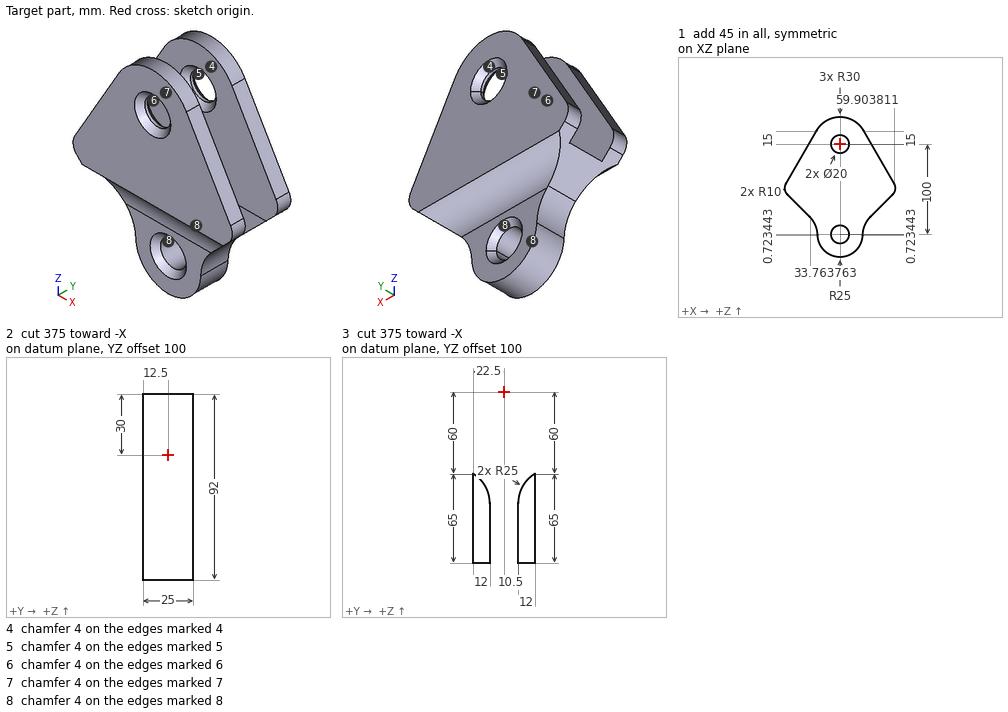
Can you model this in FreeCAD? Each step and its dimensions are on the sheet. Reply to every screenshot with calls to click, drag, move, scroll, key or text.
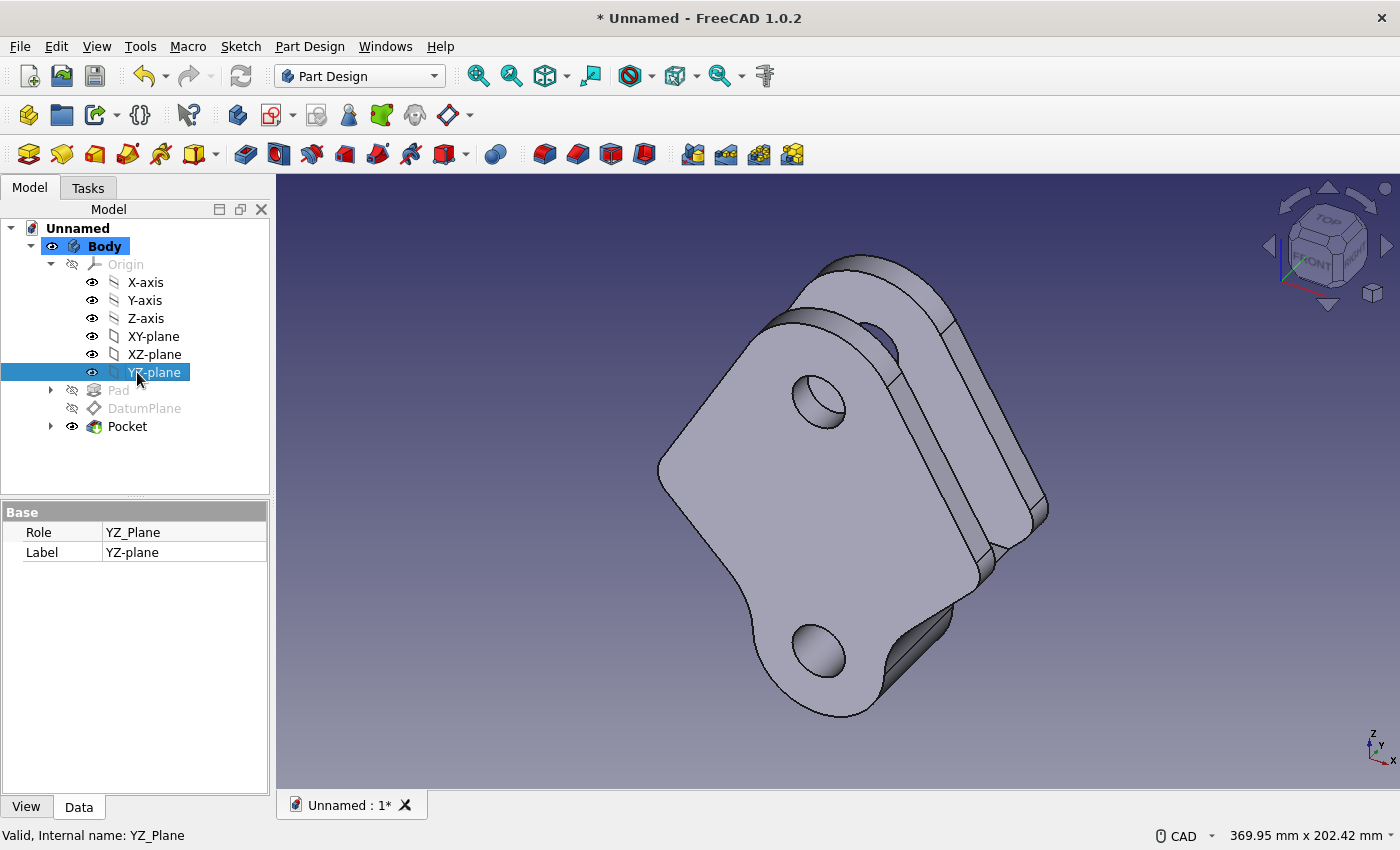
click(448, 116)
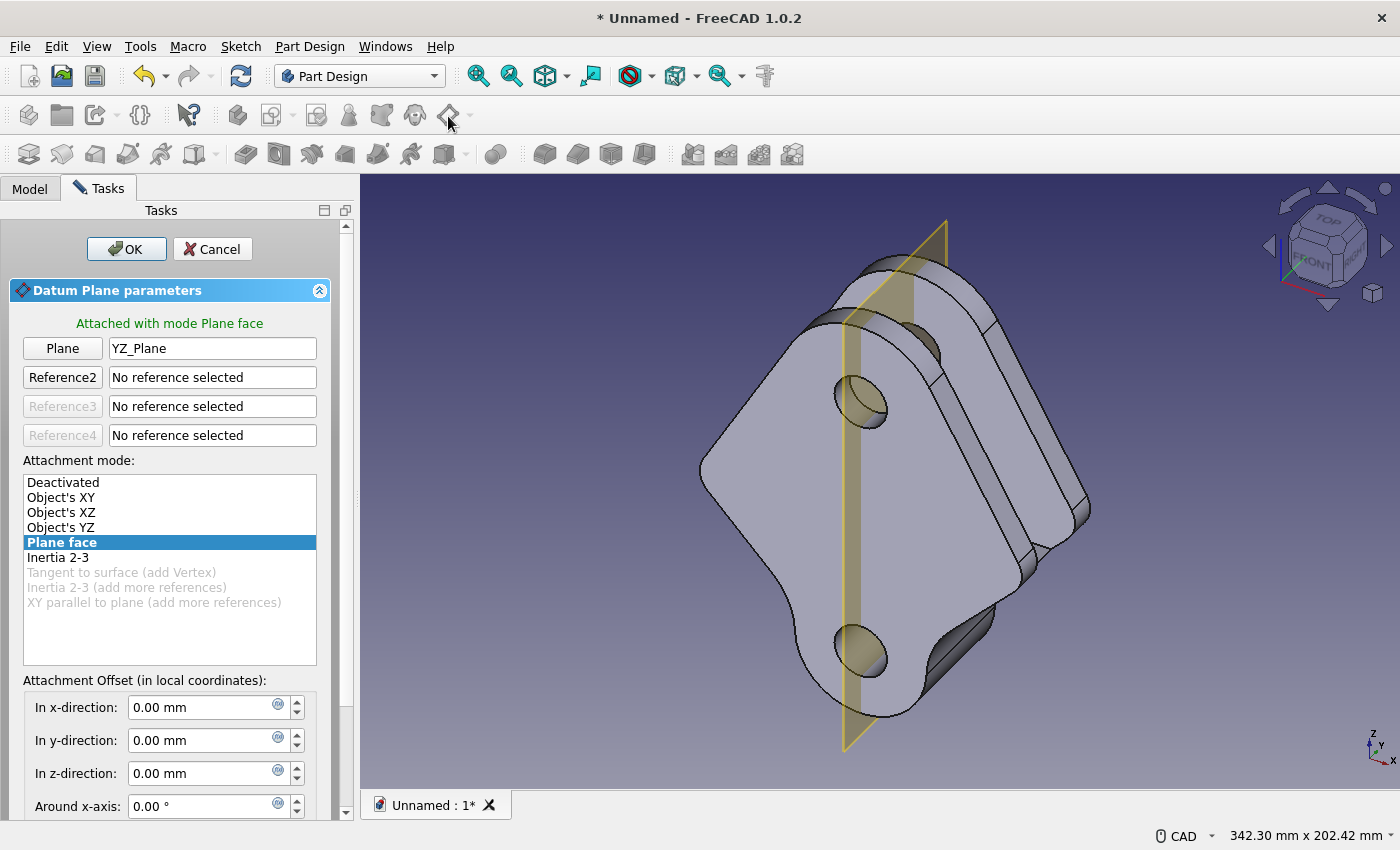
triple_click(210, 774)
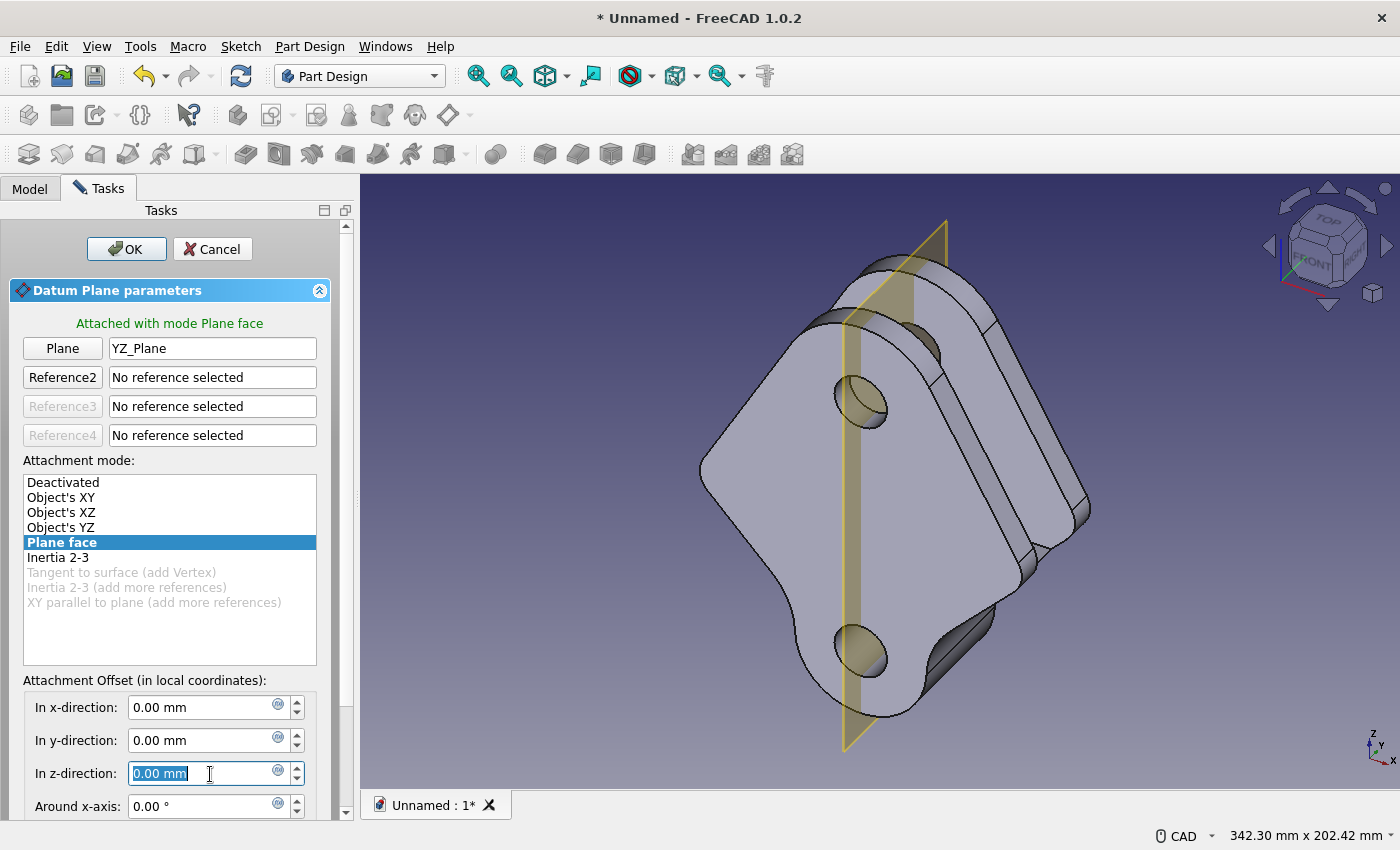
text(100)
key(Tab)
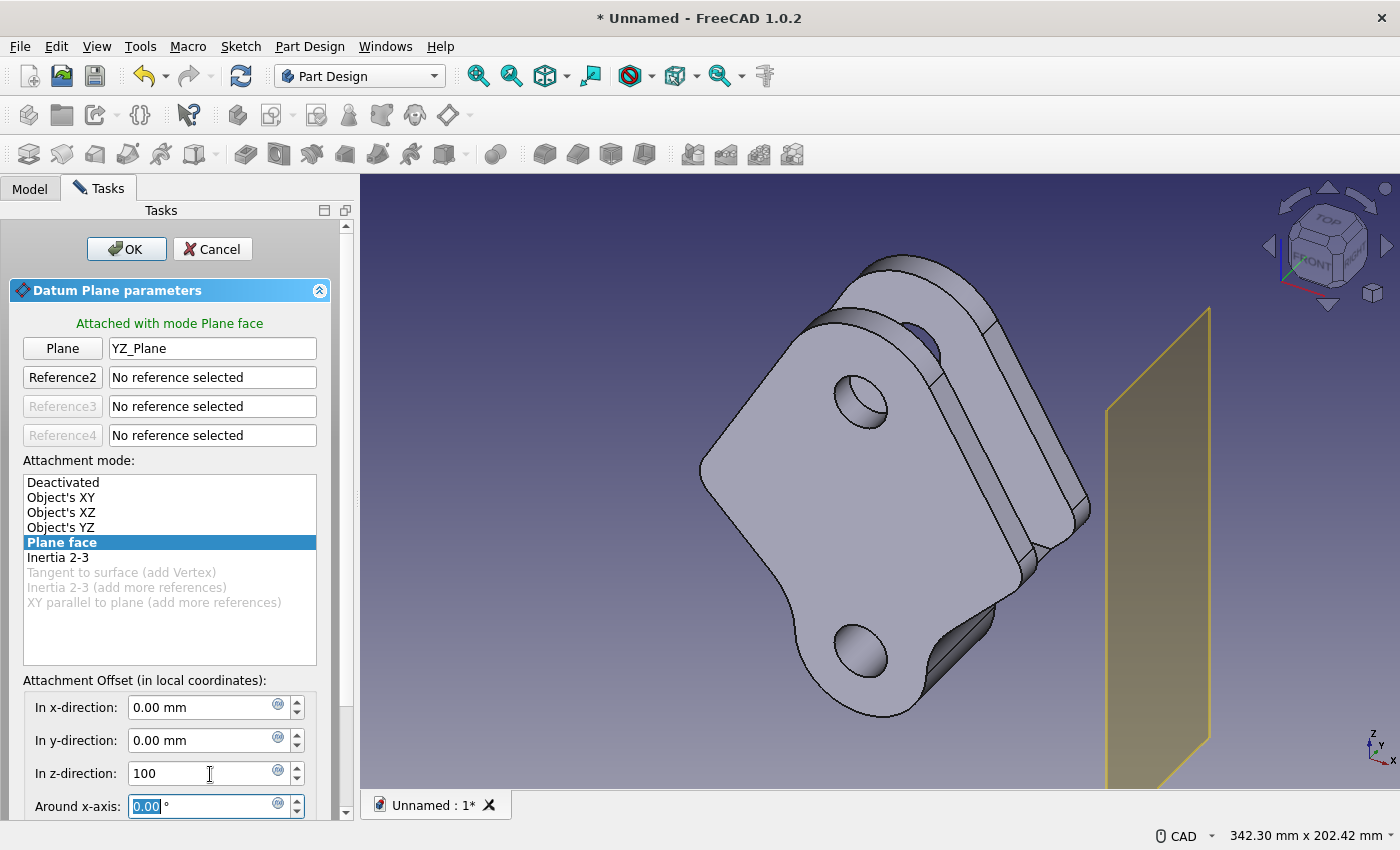
click(127, 249)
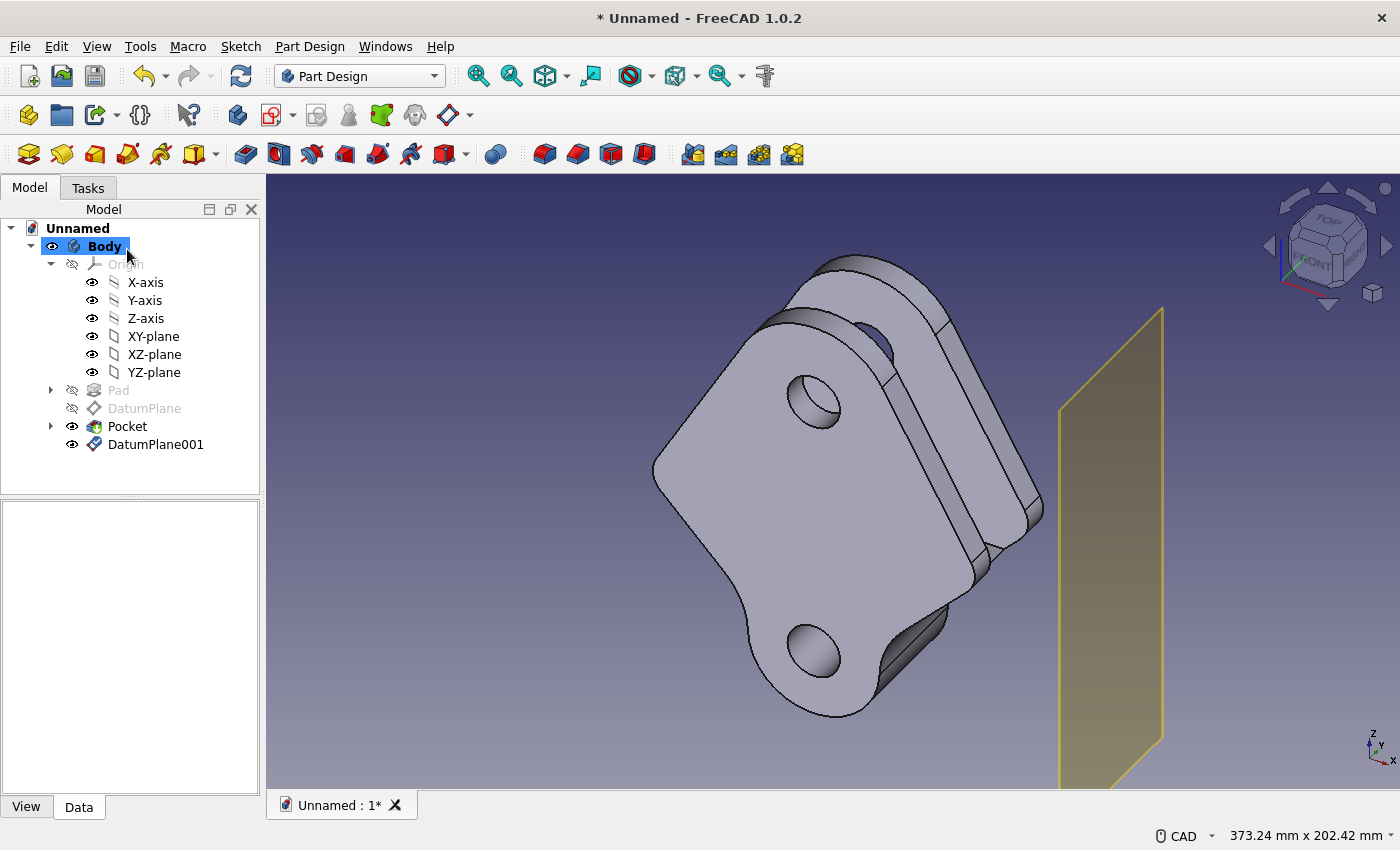
click(117, 444)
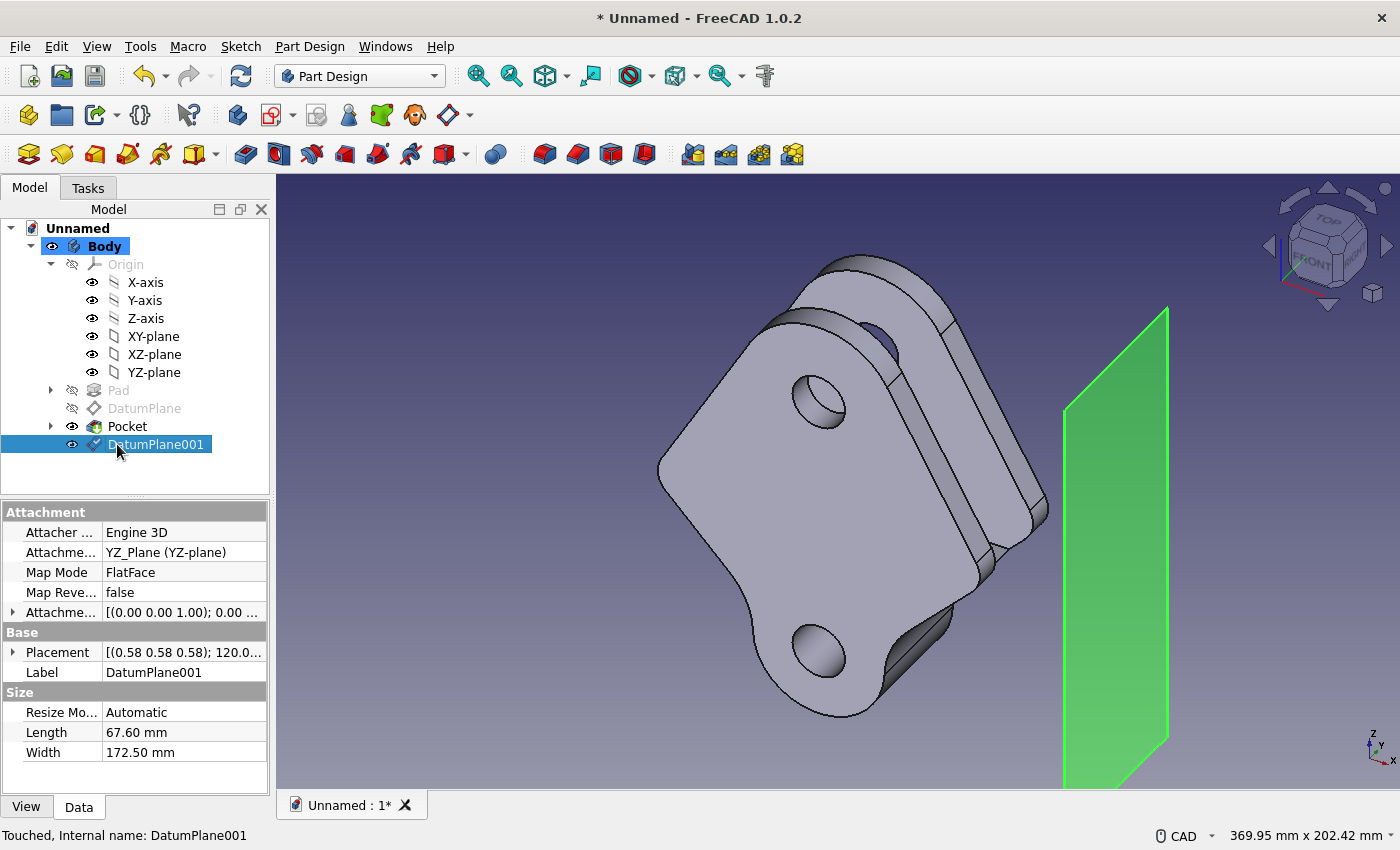
click(270, 116)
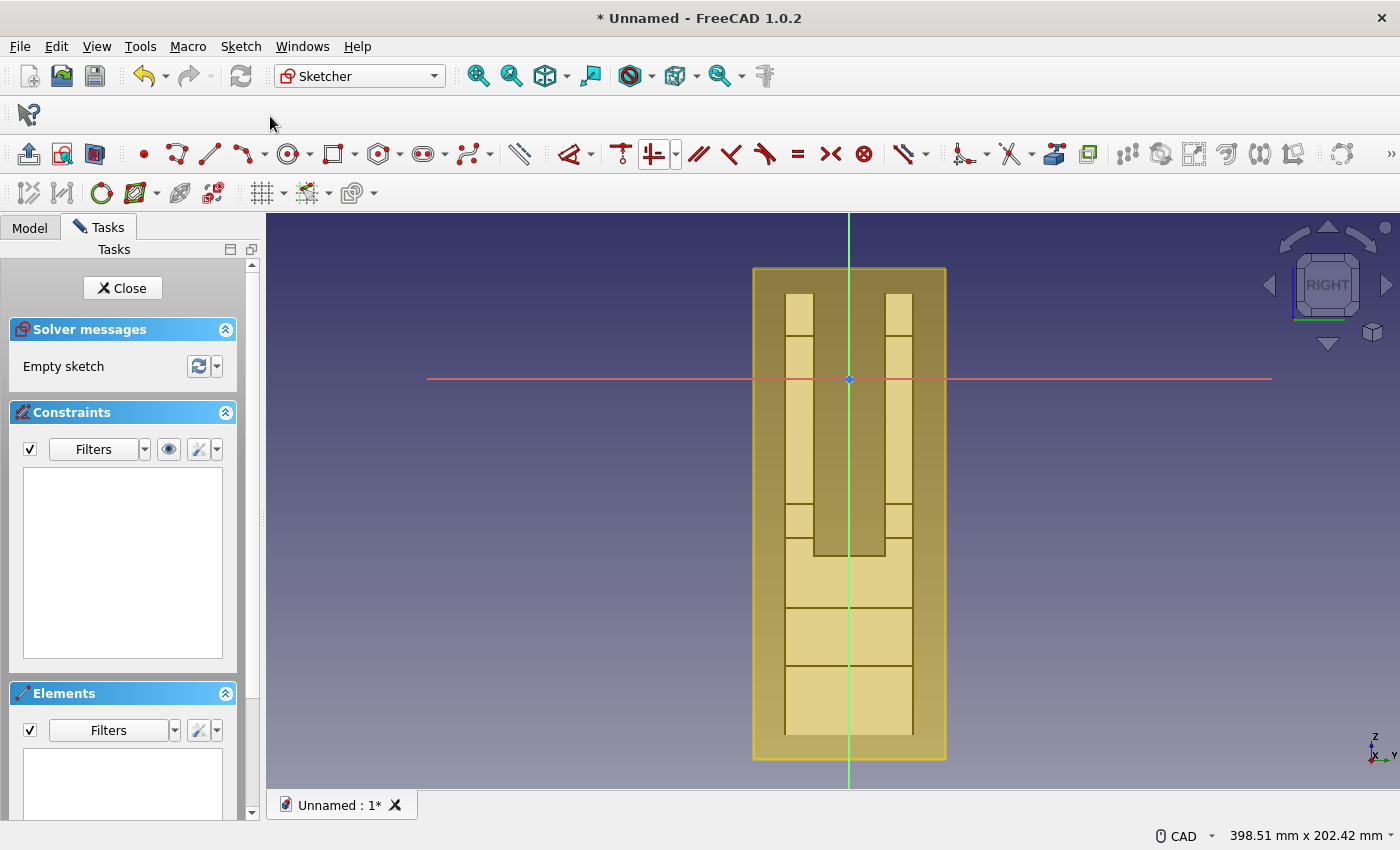
click(177, 154)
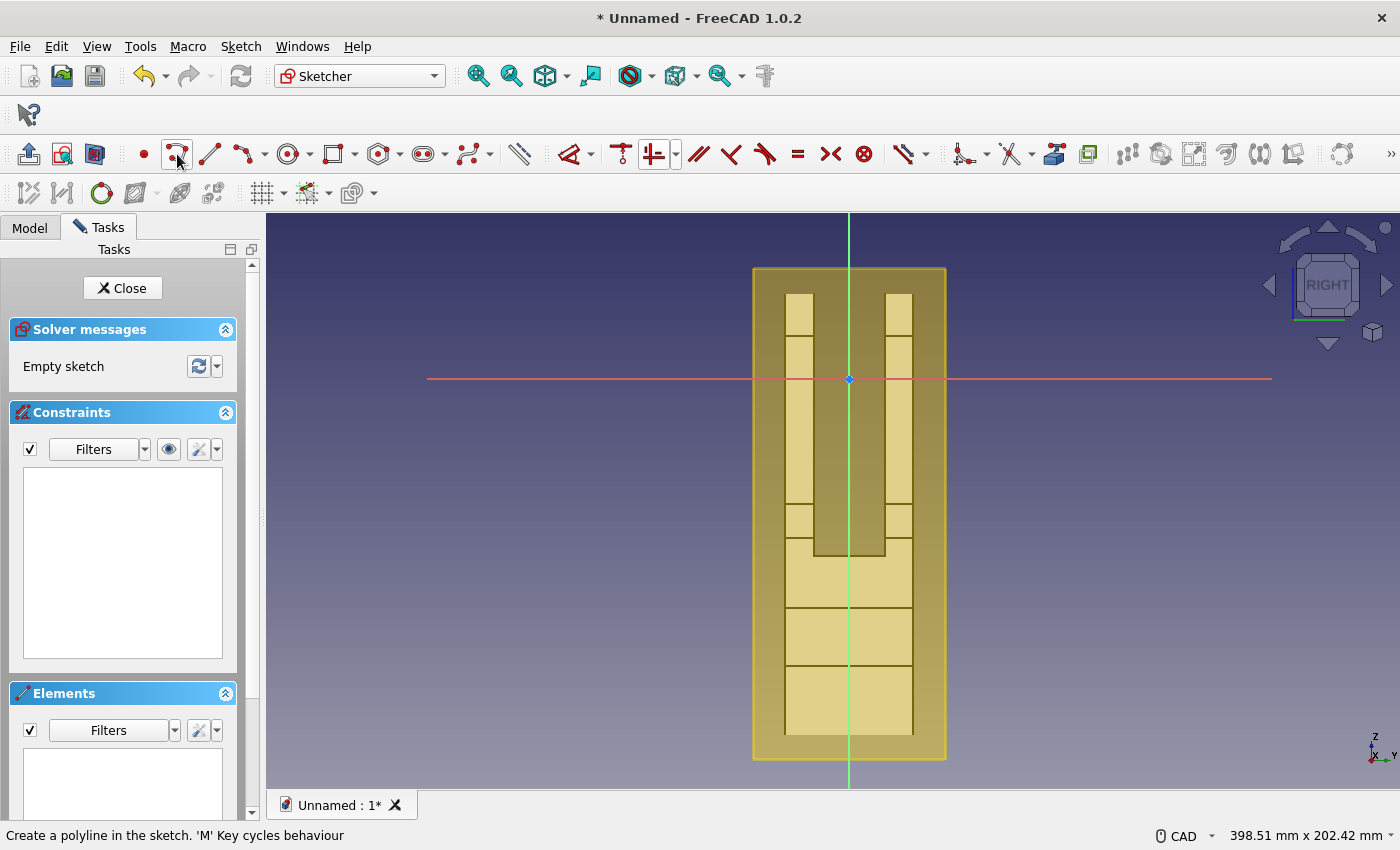
click(879, 611)
click(879, 735)
click(913, 735)
click(913, 550)
right_click(913, 550)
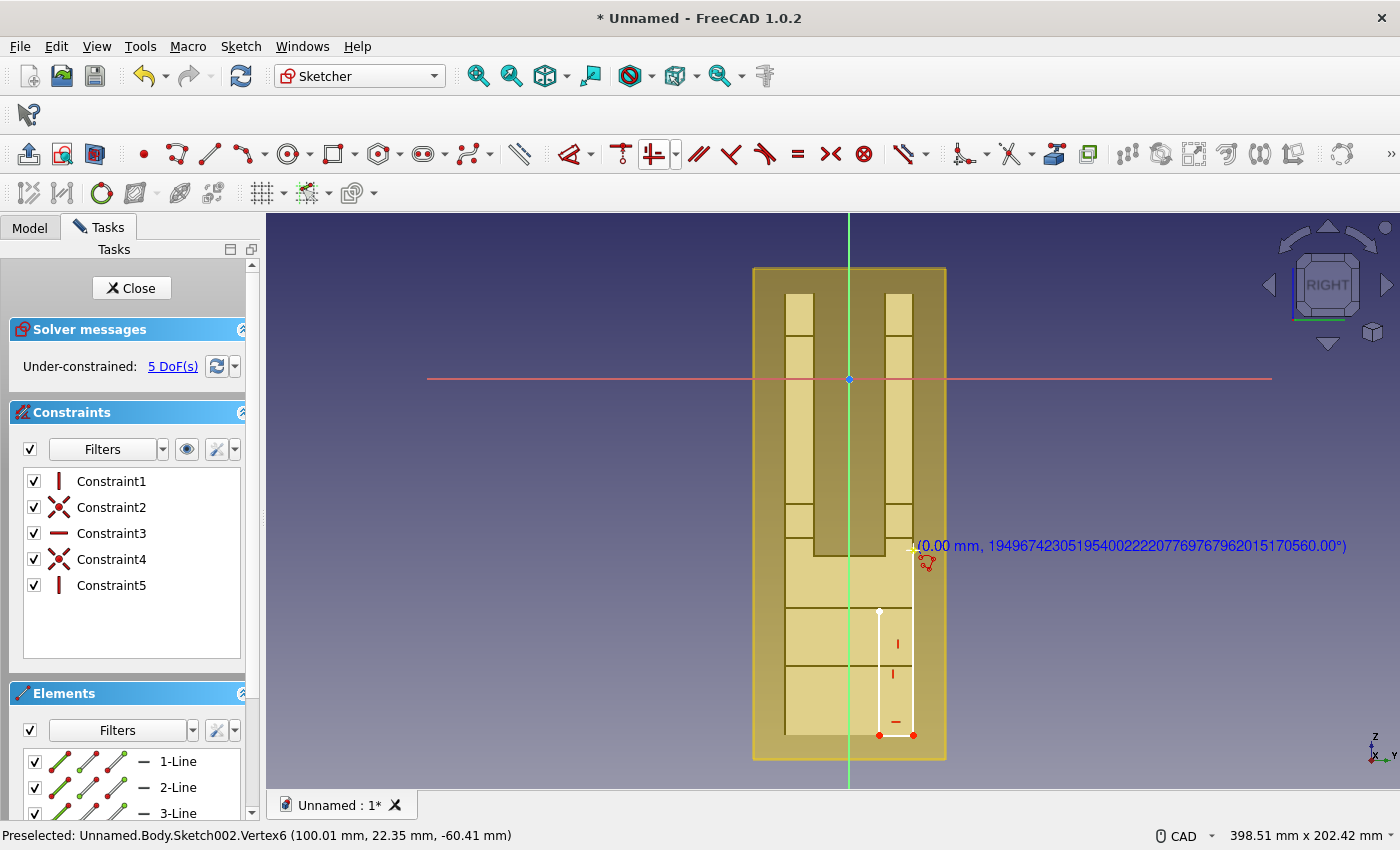
key(g)
key(3)
key(a)